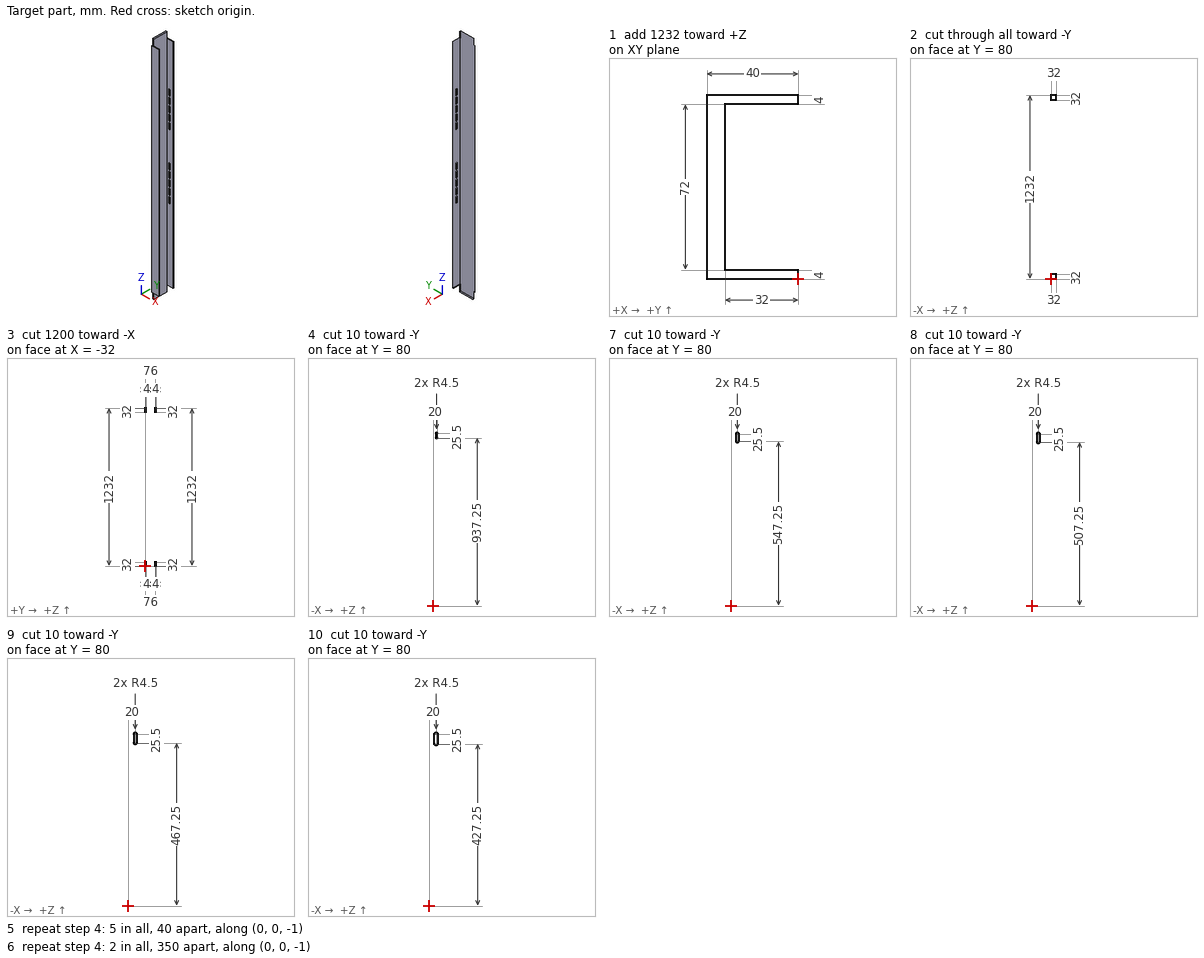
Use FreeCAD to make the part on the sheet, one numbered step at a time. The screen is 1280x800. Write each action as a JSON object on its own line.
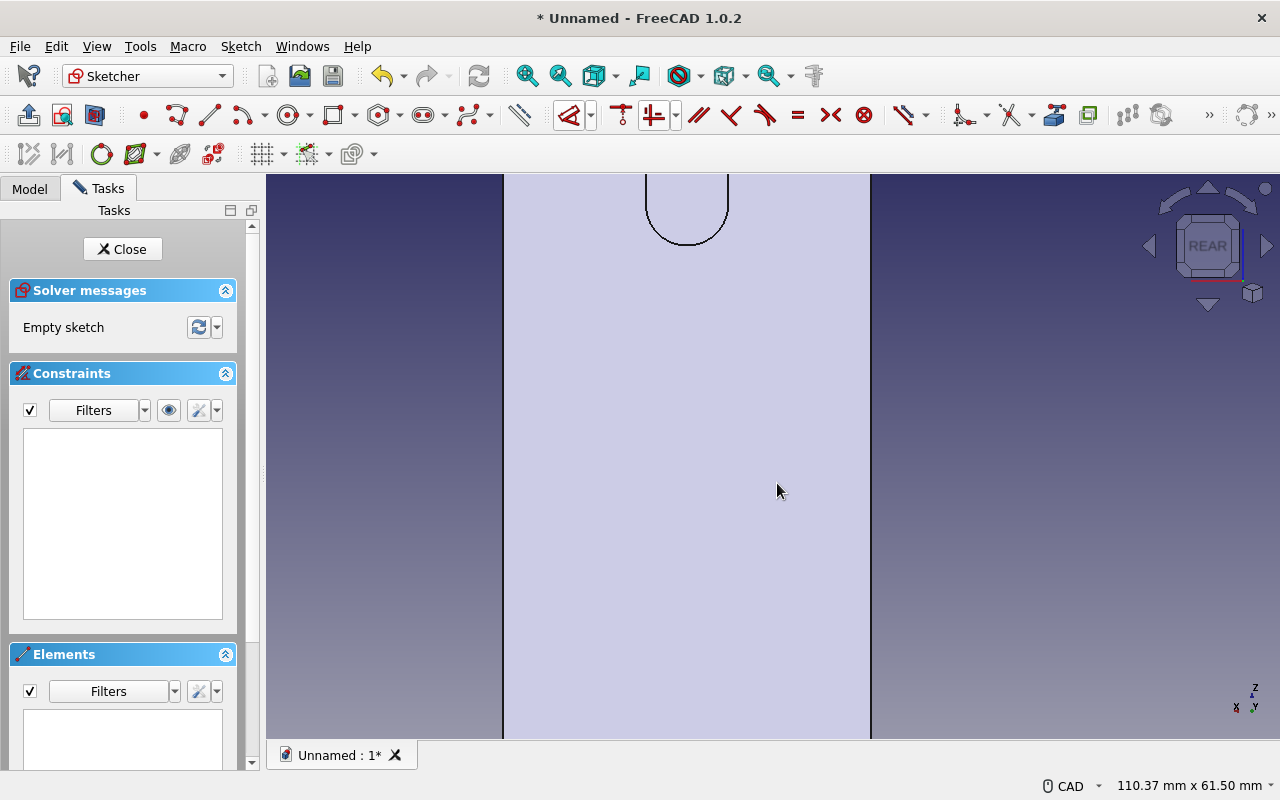
{"action": "left_click", "coordinate": [422, 116]}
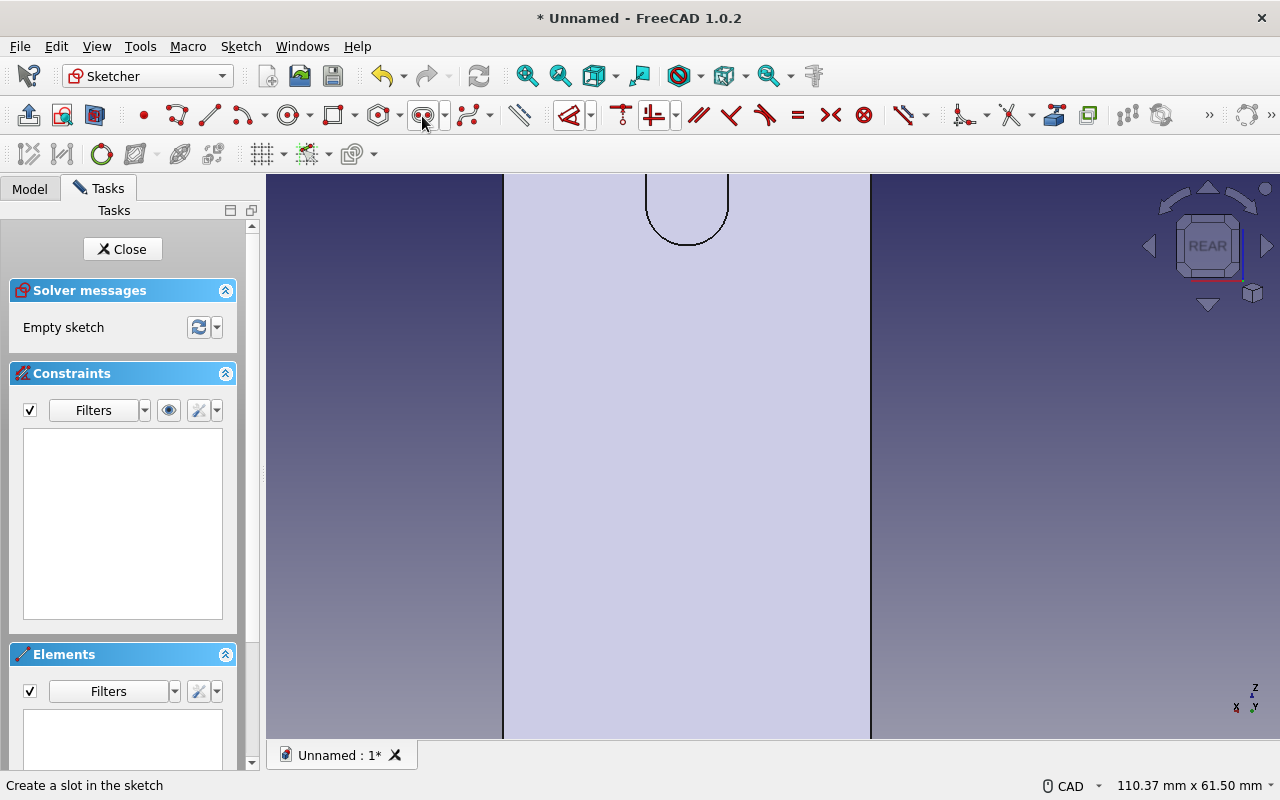
{"action": "left_click", "coordinate": [687, 572]}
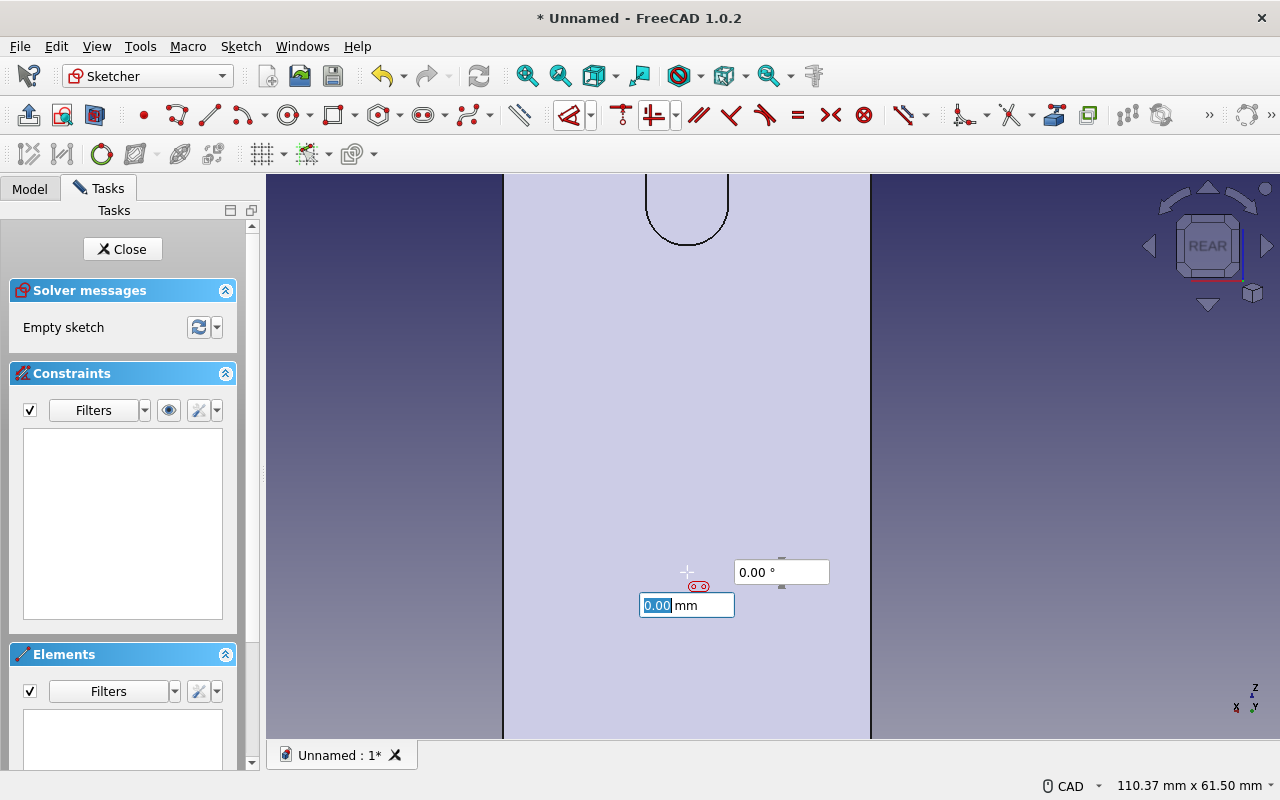
{"action": "left_click", "coordinate": [687, 338]}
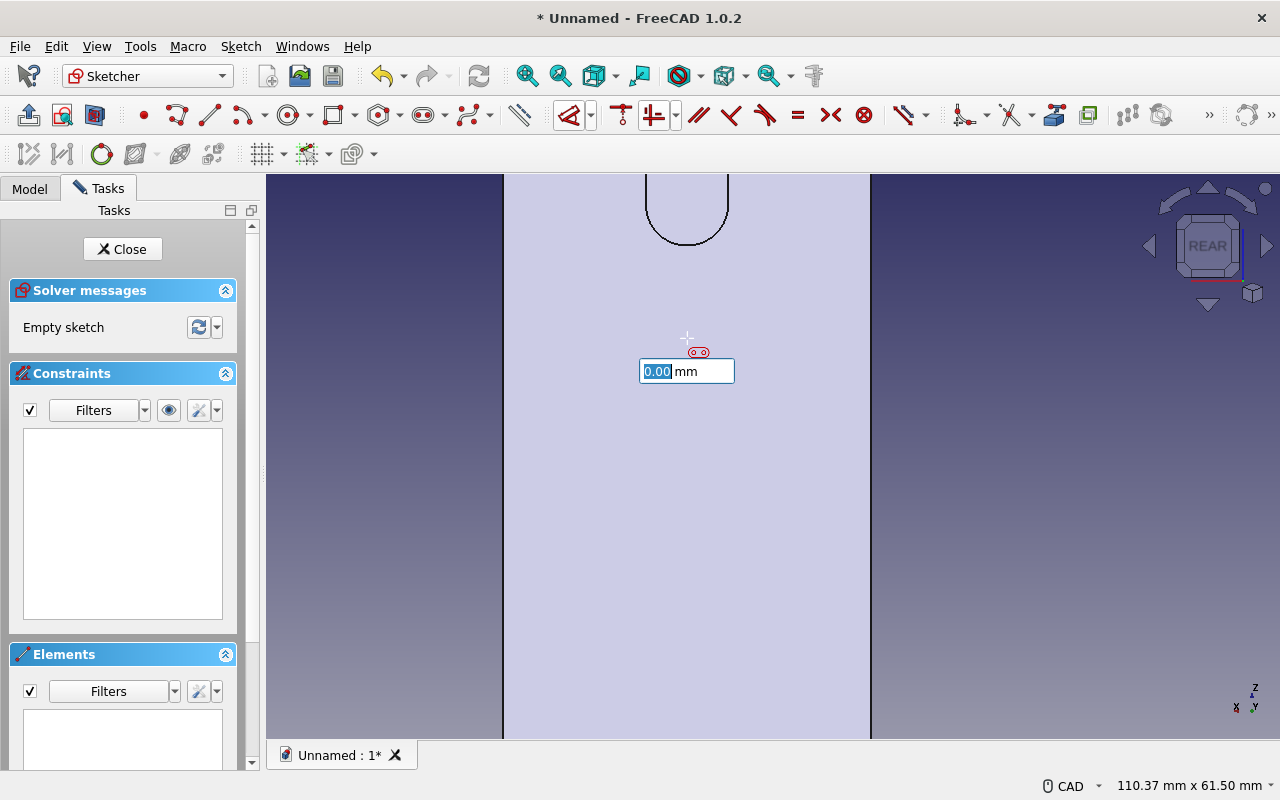
{"action": "left_click", "coordinate": [728, 455]}
{"action": "key", "text": "Escape"}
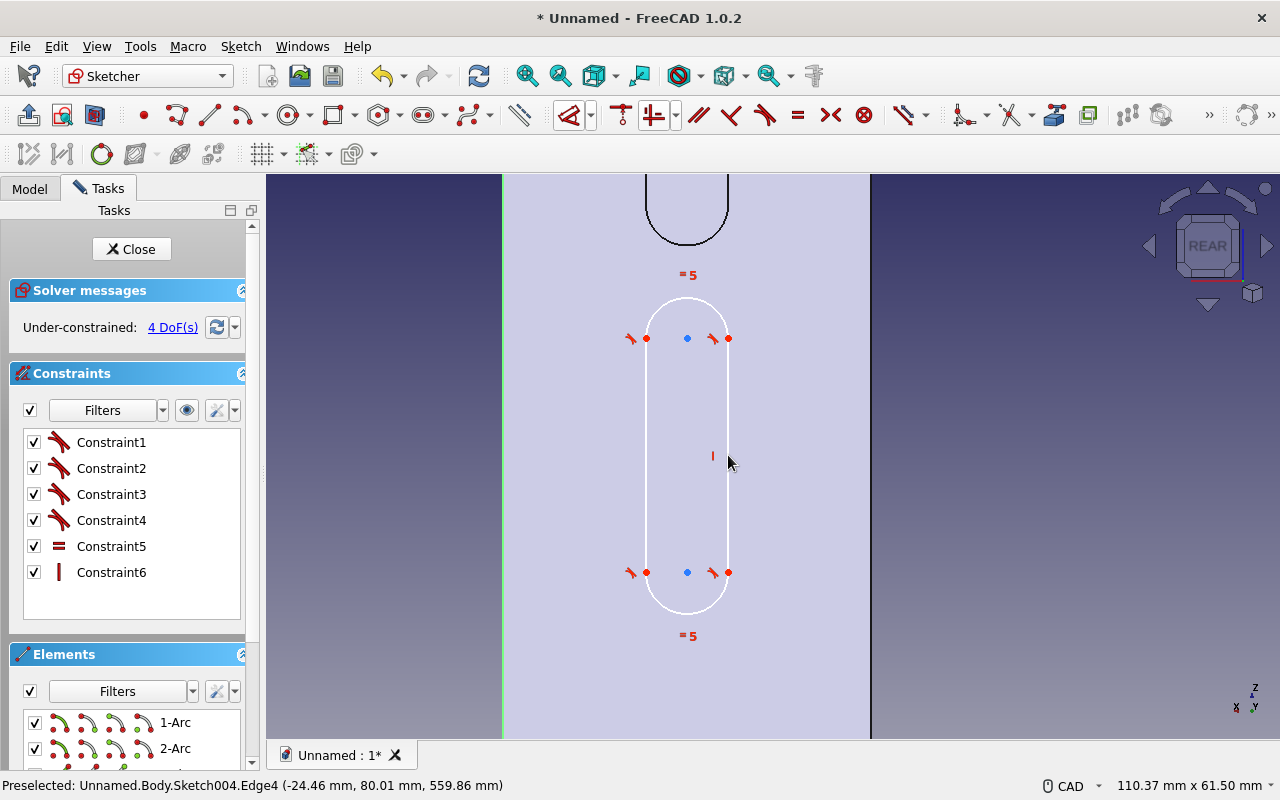
{"action": "left_click", "coordinate": [663, 606]}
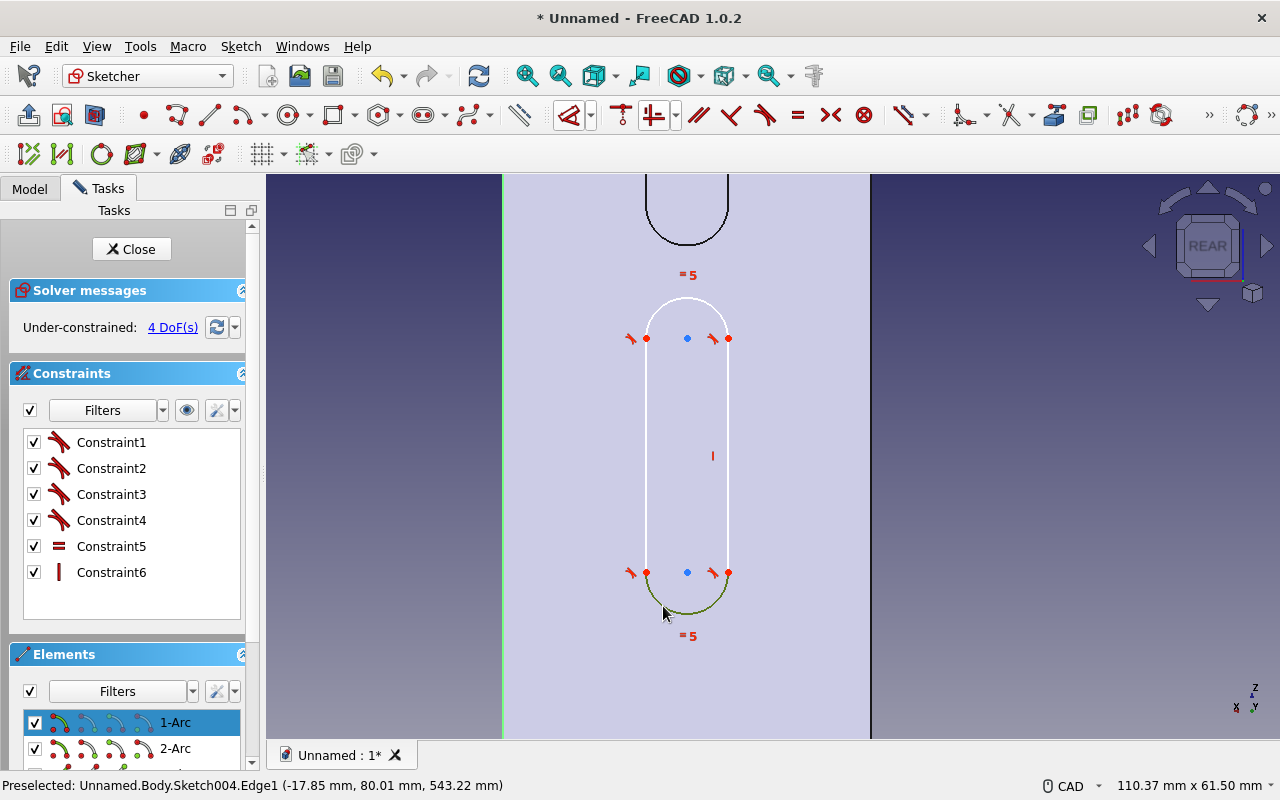
{"action": "left_click", "coordinate": [590, 116]}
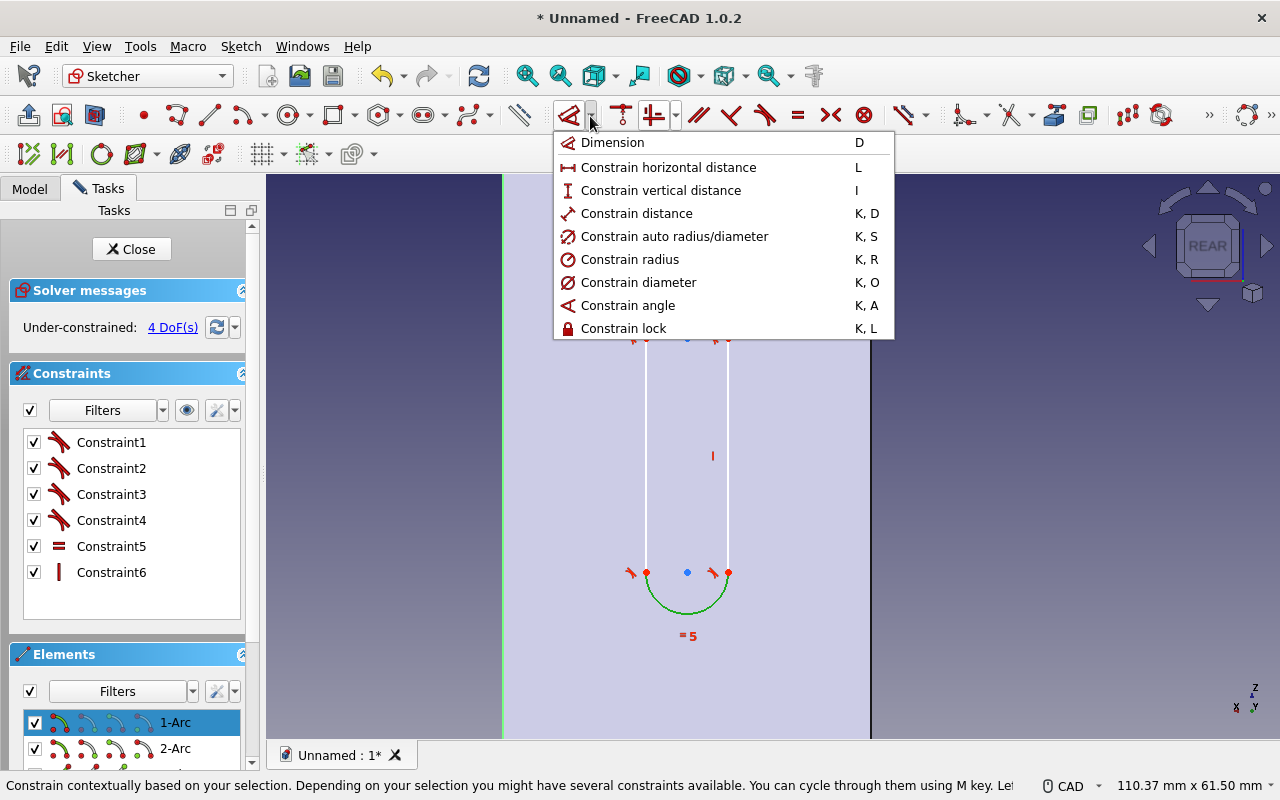
{"action": "left_click", "coordinate": [724, 260]}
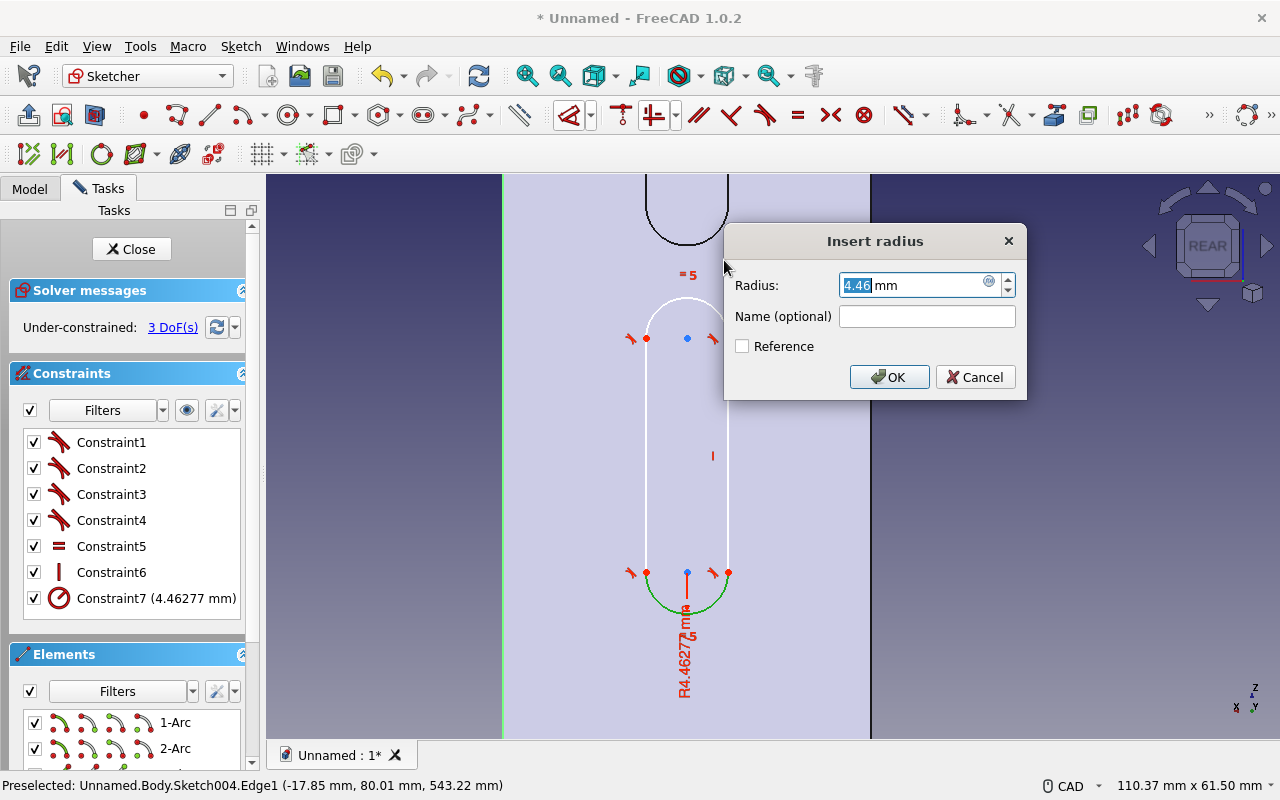
{"action": "type", "text": "4.5"}
{"action": "key", "text": "Return"}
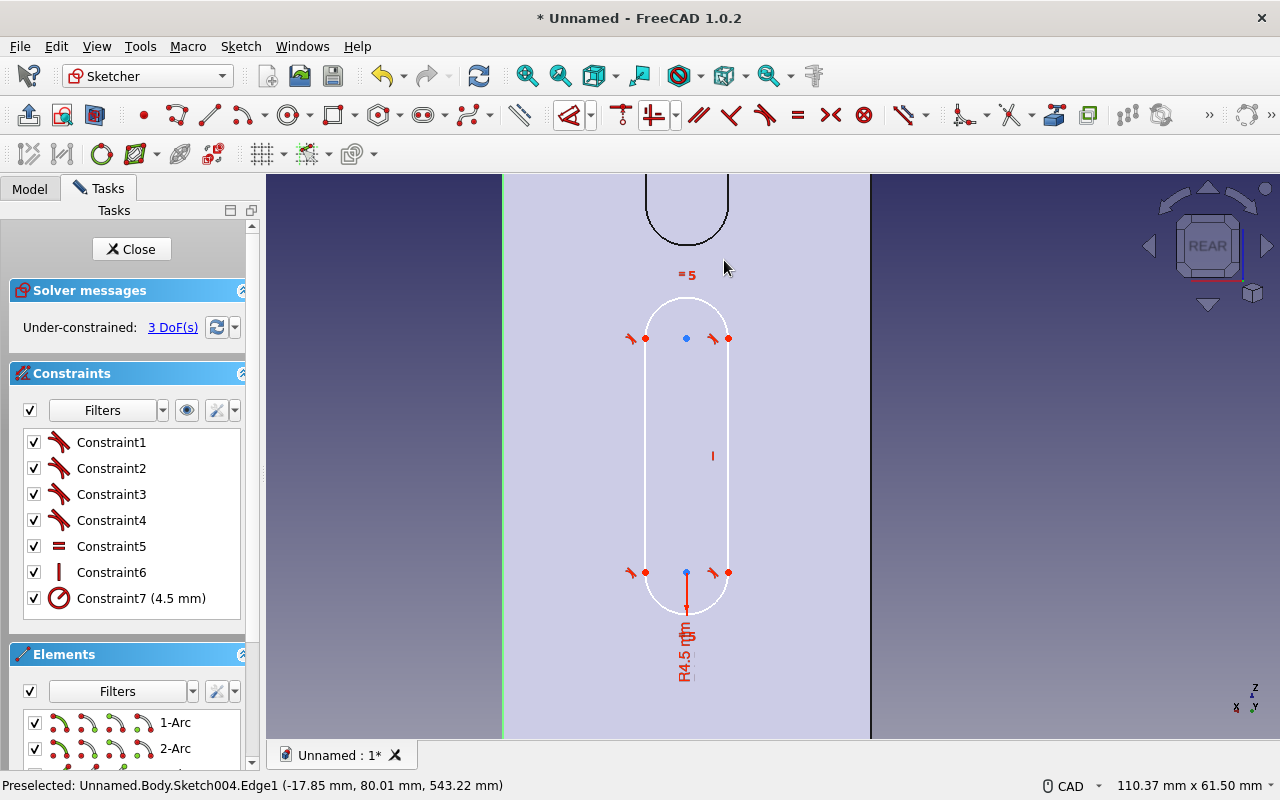
{"action": "left_click", "coordinate": [687, 573]}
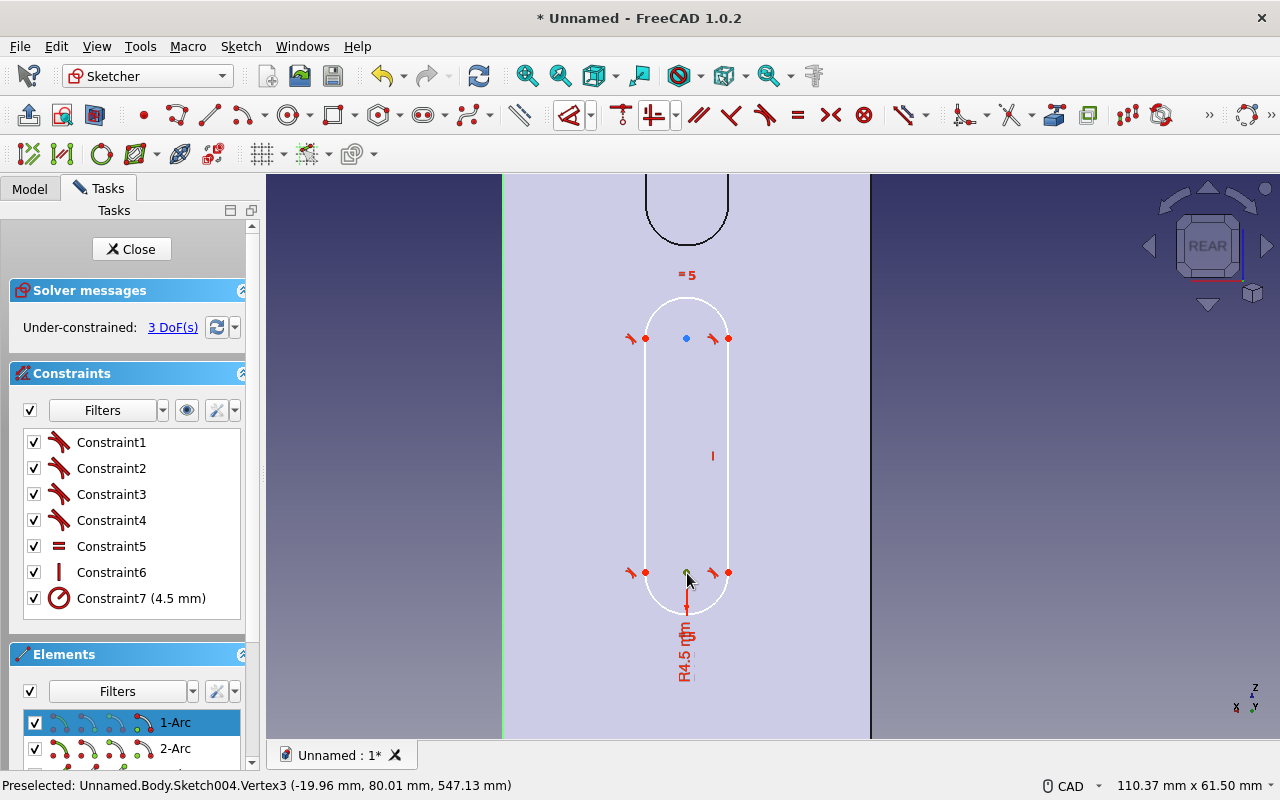
{"action": "key", "text": "l"}